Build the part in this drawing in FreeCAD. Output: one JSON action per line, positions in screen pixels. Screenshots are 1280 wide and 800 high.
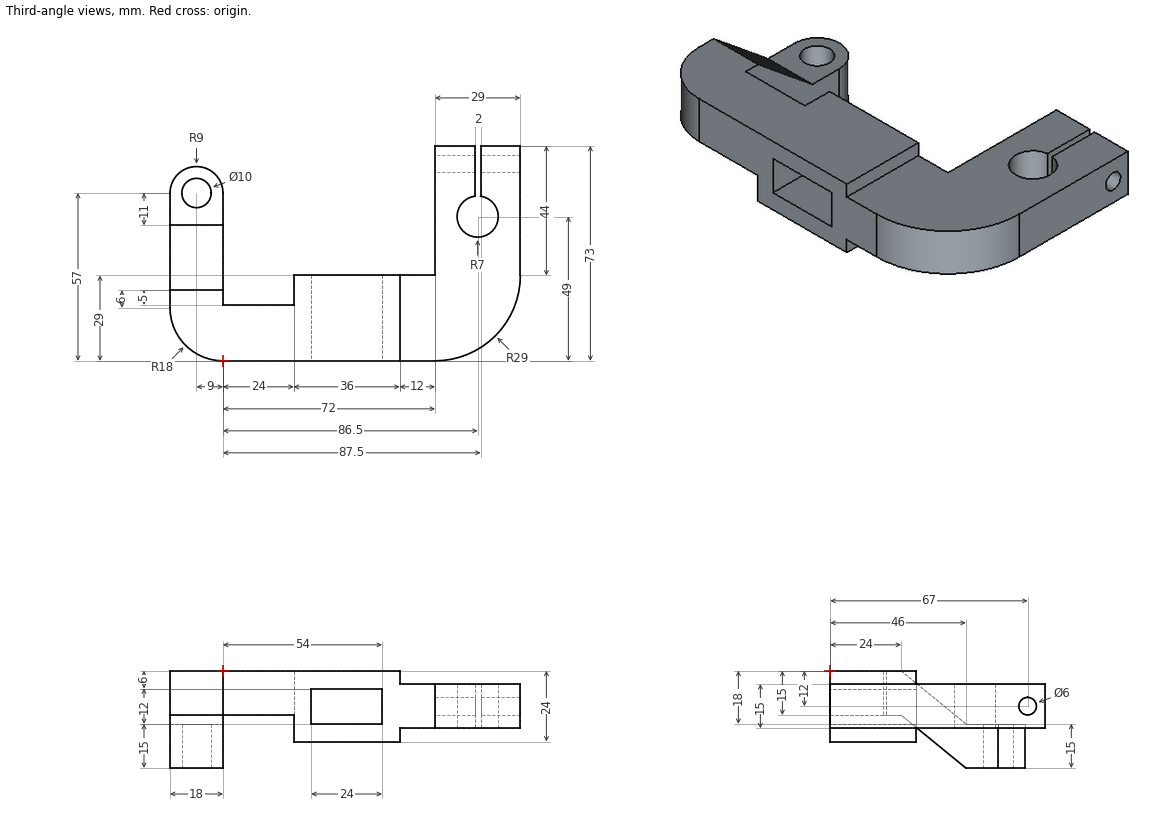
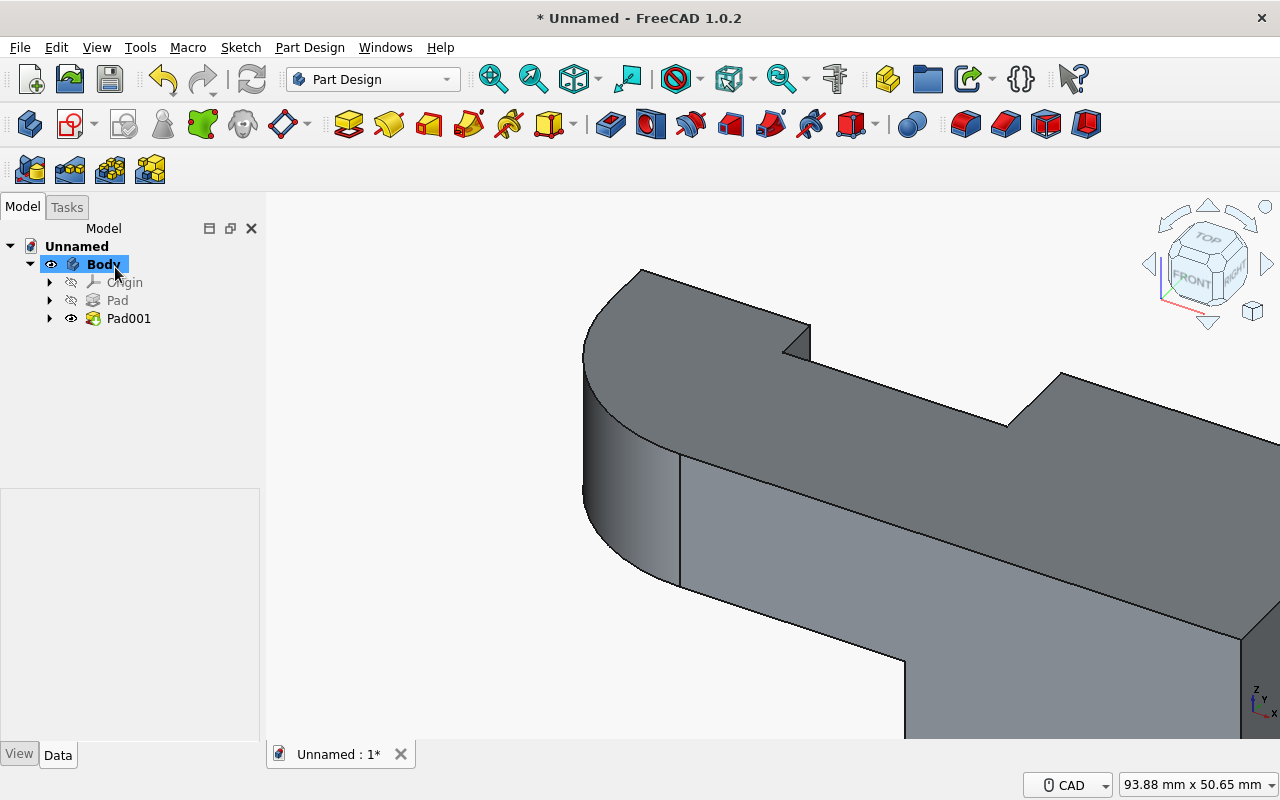
{"action": "left_click", "coordinate": [494, 80]}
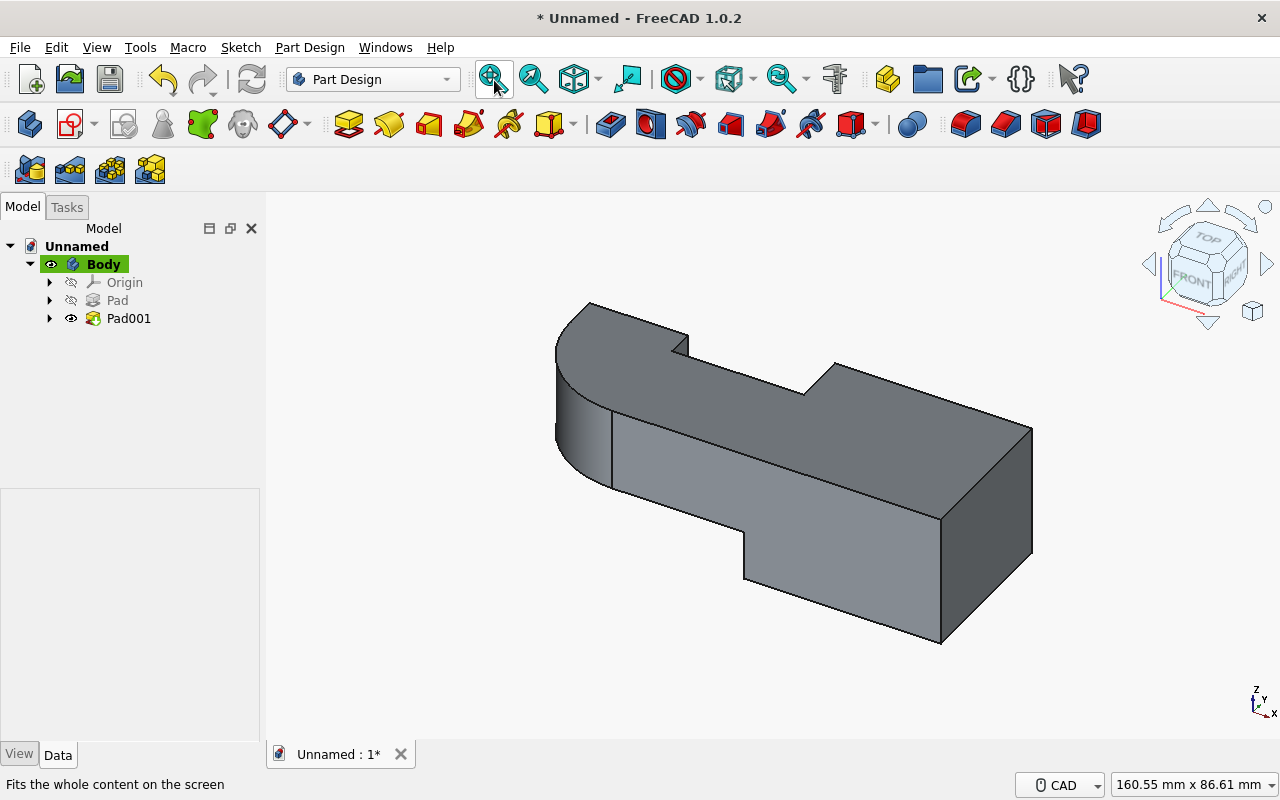
{"action": "left_click", "coordinate": [50, 282]}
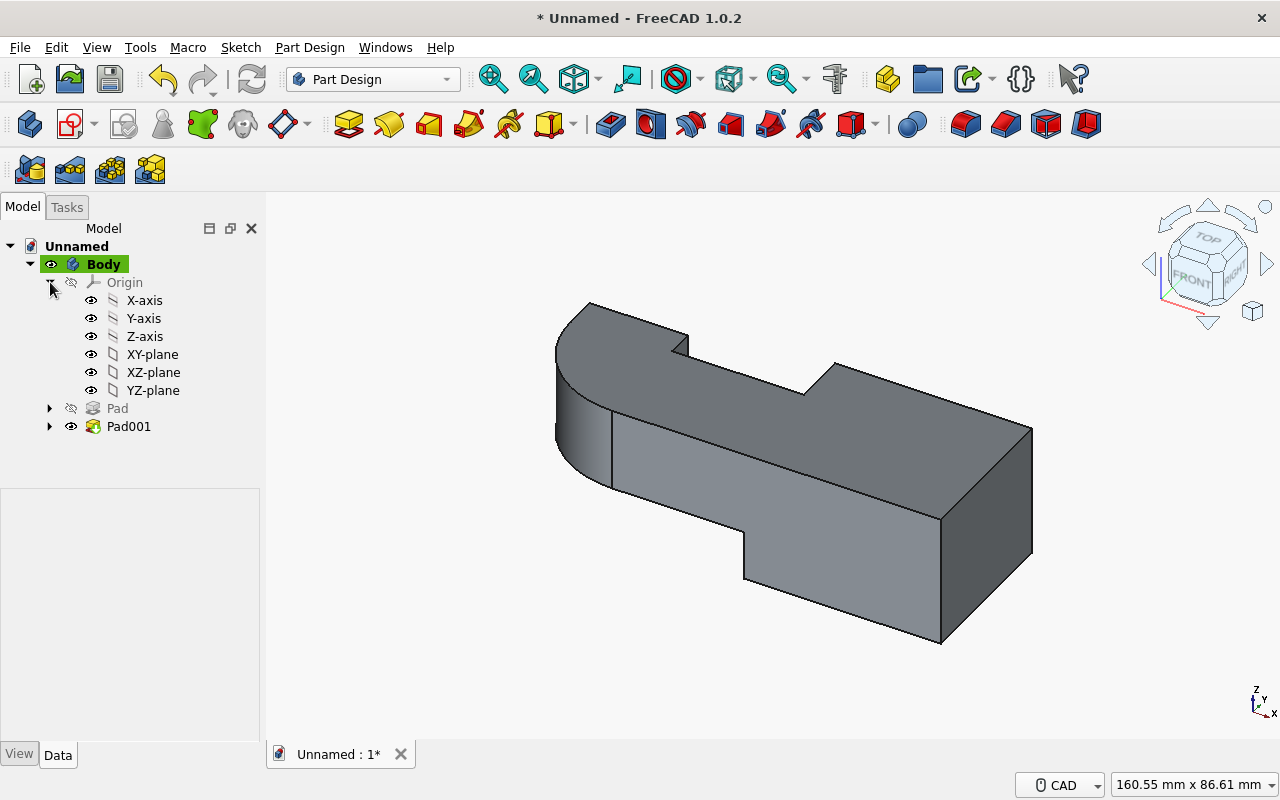
{"action": "left_click", "coordinate": [136, 354]}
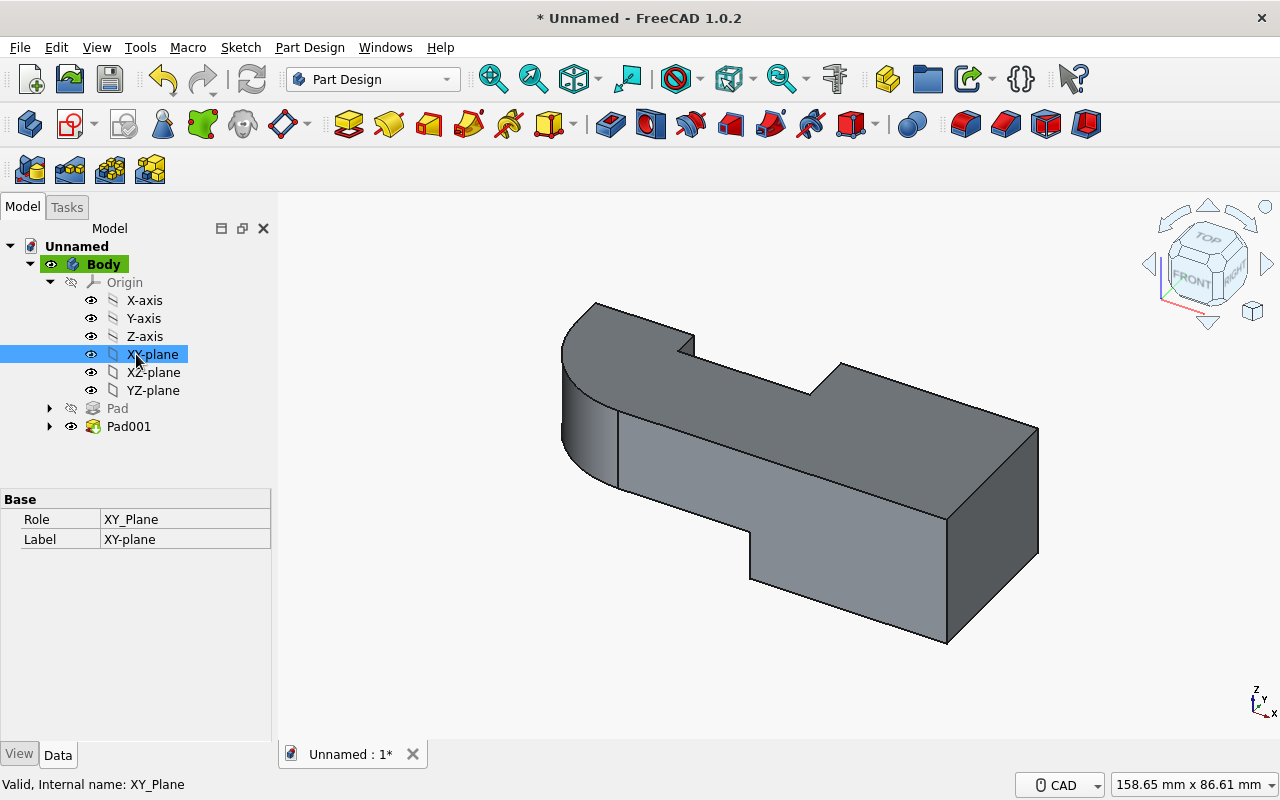
{"action": "left_click", "coordinate": [284, 124]}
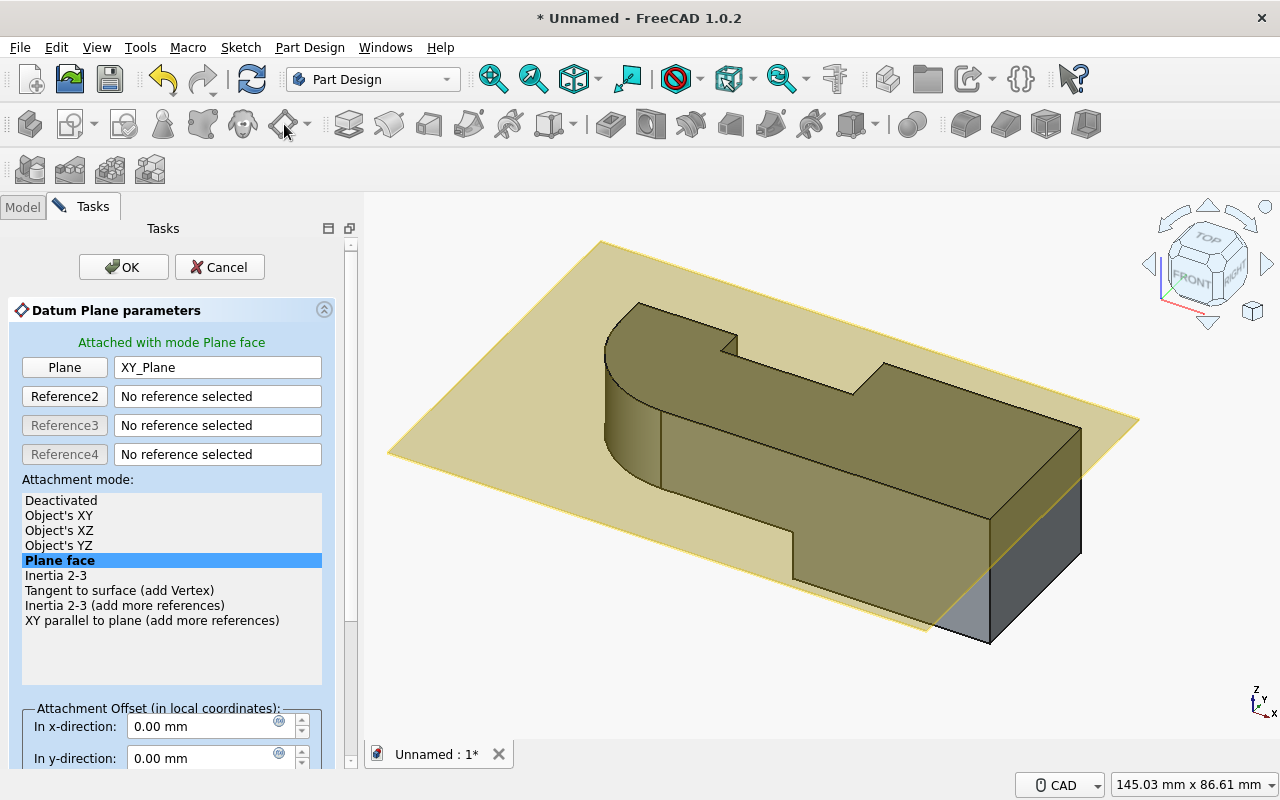
{"action": "scroll", "coordinate": [351, 503], "scroll_direction": "down", "scroll_amount": 2}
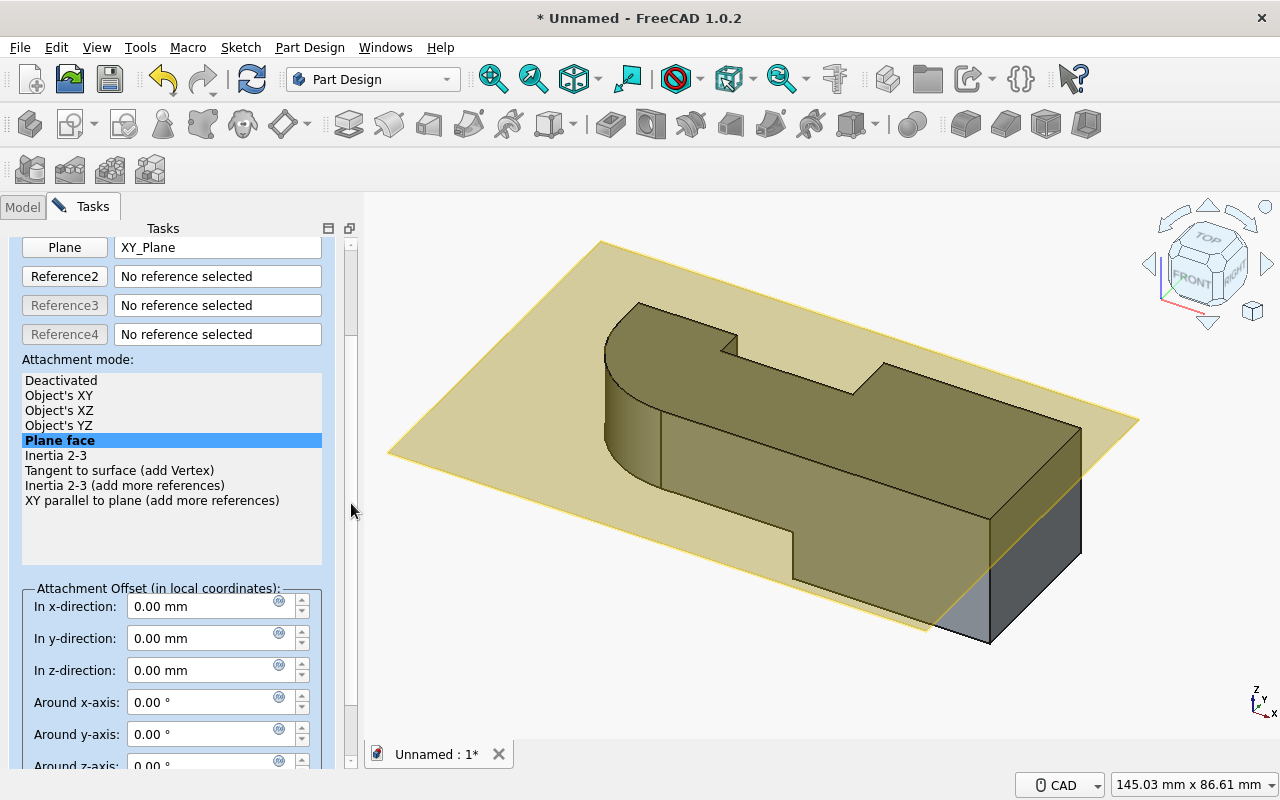
{"action": "triple_click", "coordinate": [210, 670]}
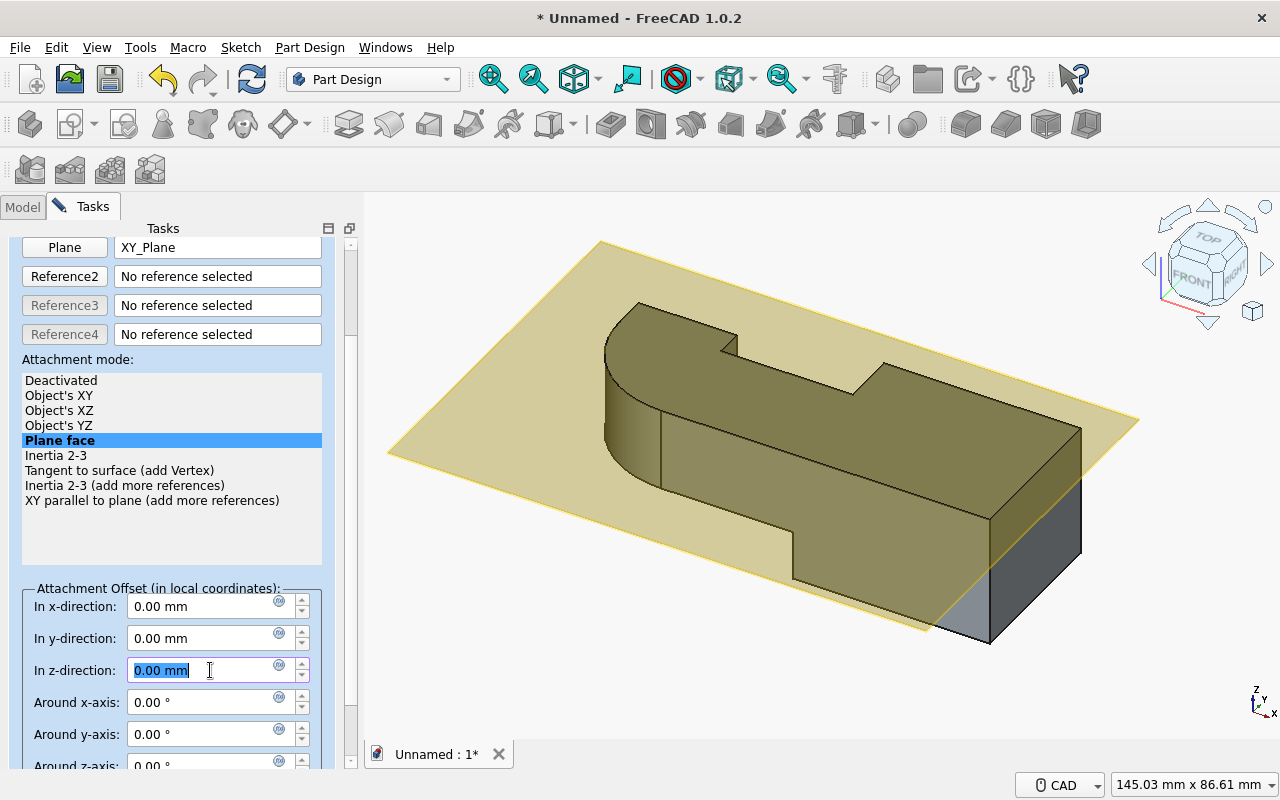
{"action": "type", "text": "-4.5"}
{"action": "key", "text": "Tab"}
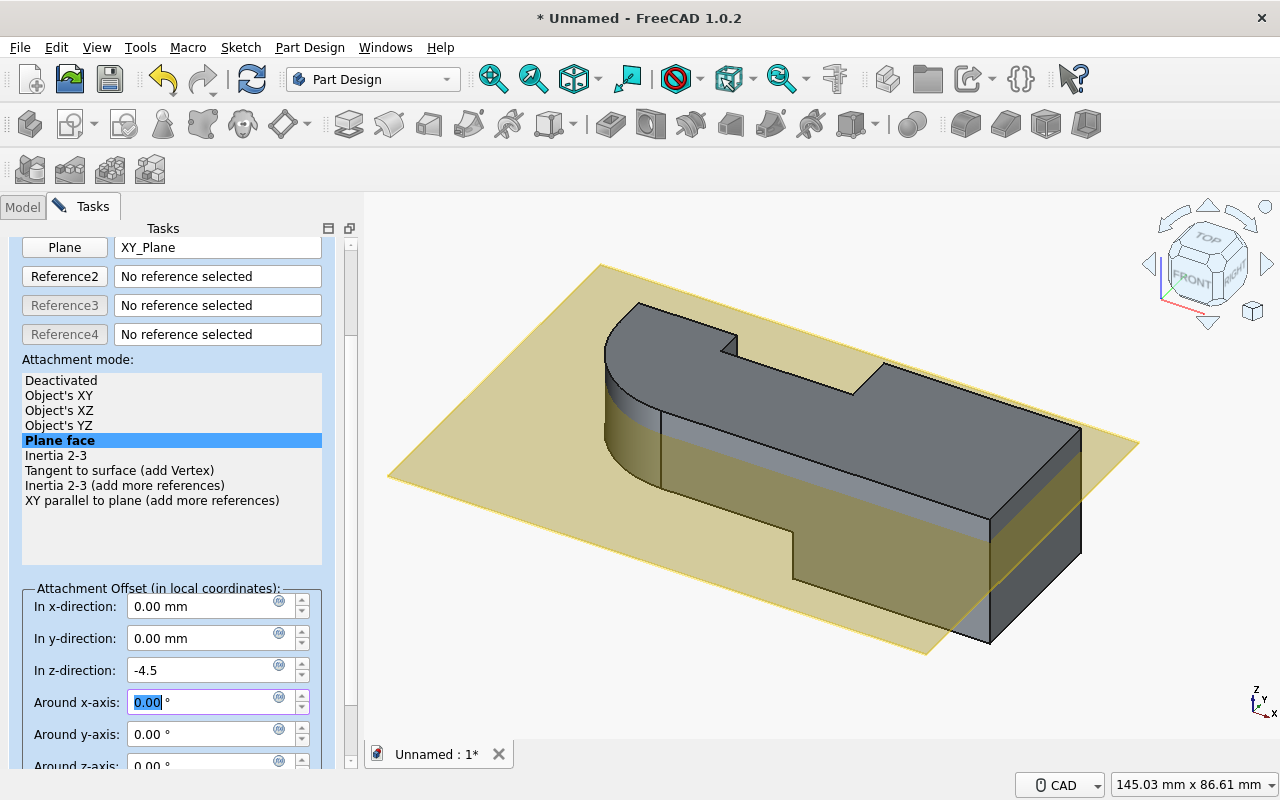
{"action": "scroll", "coordinate": [351, 503], "scroll_direction": "up", "scroll_amount": 3}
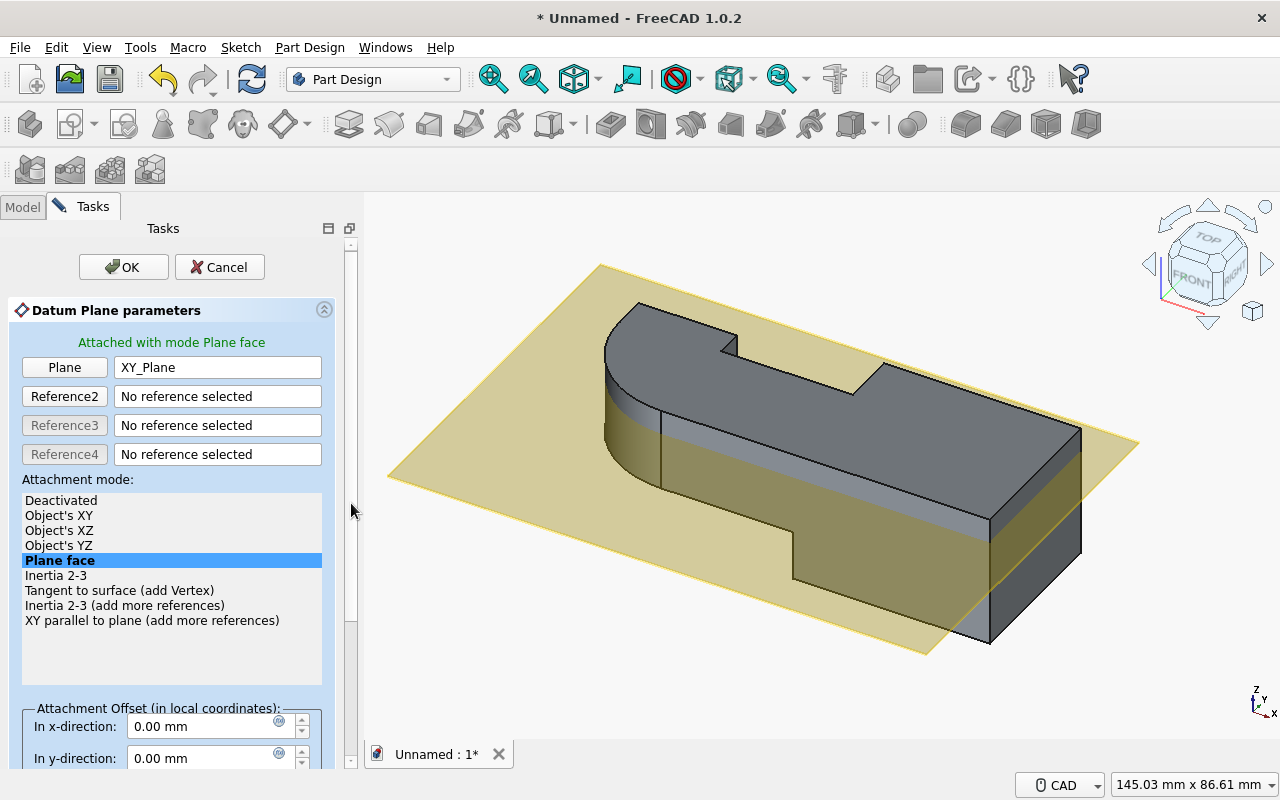
{"action": "left_click", "coordinate": [124, 267]}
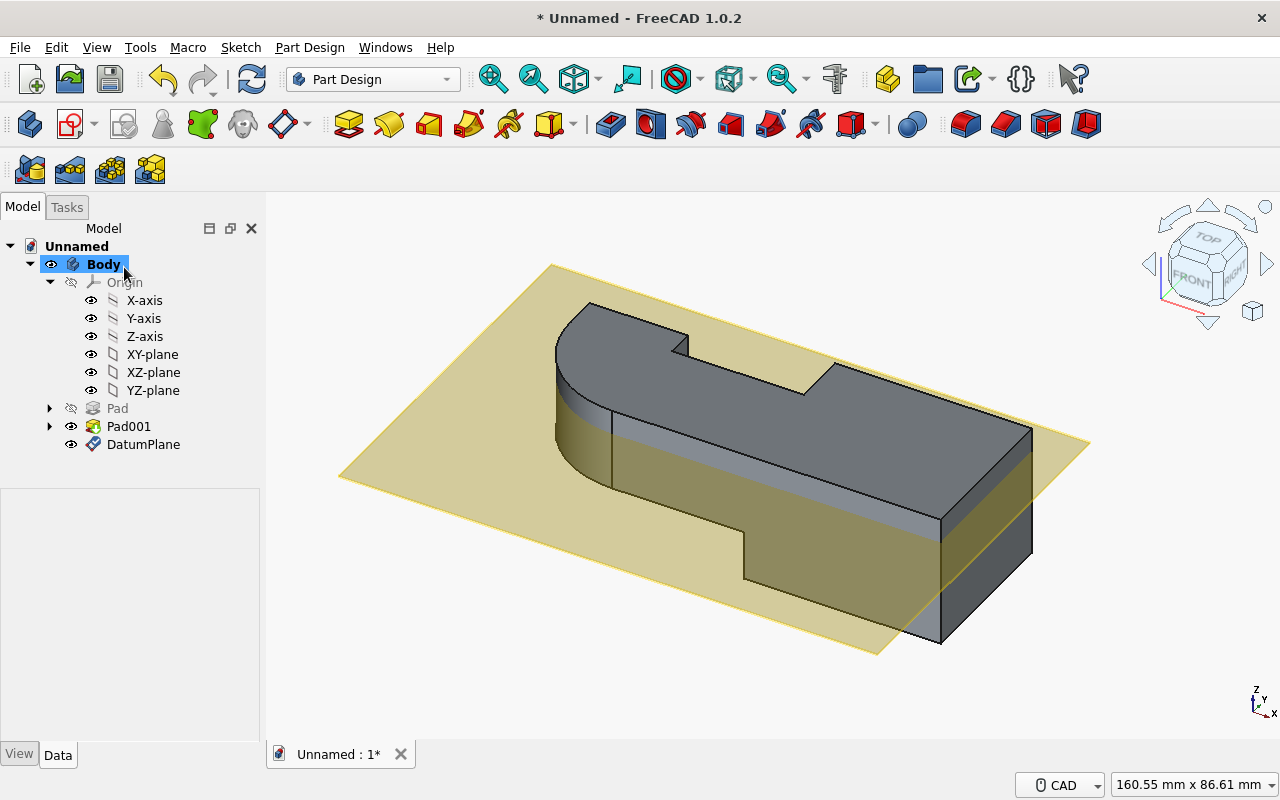
{"action": "left_click", "coordinate": [116, 444]}